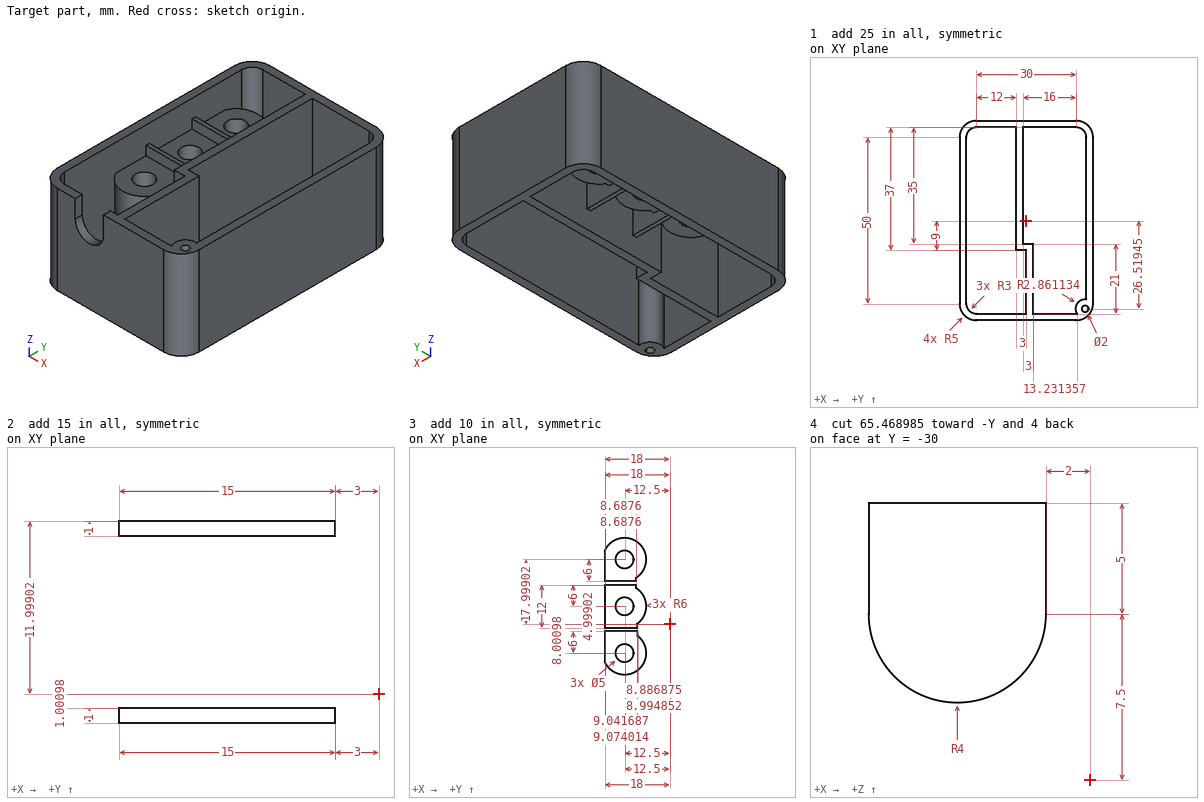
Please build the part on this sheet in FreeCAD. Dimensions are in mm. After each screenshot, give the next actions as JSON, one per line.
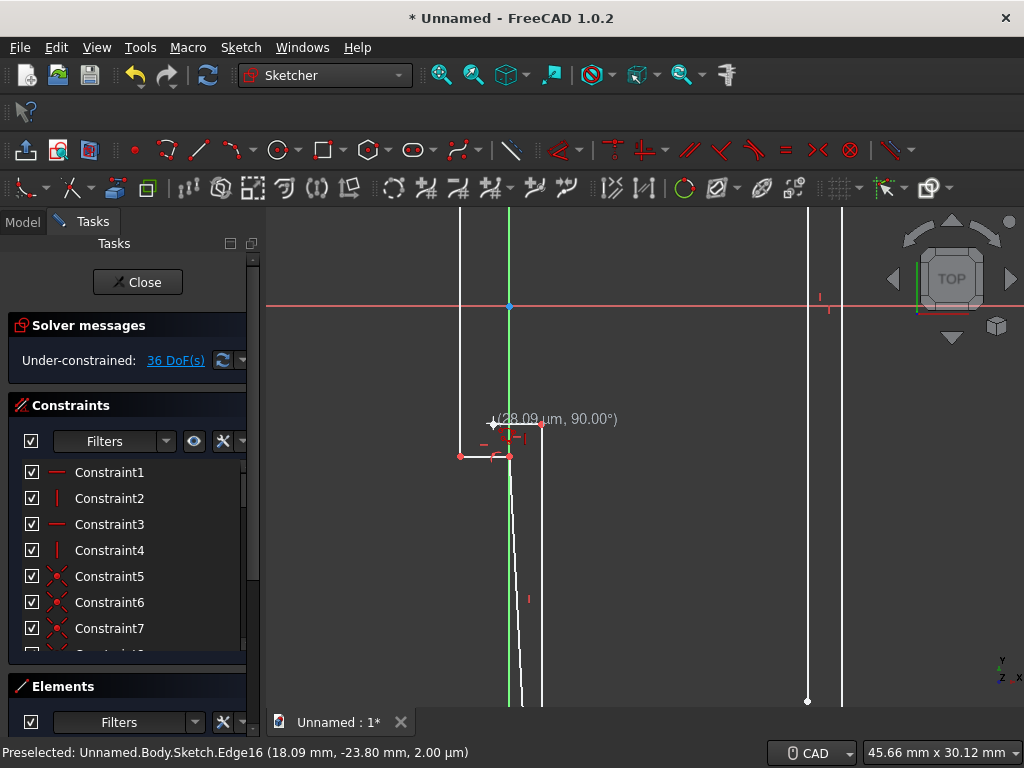
{"action": "scroll", "coordinate": [605, 522], "scroll_direction": "down", "scroll_amount": 6}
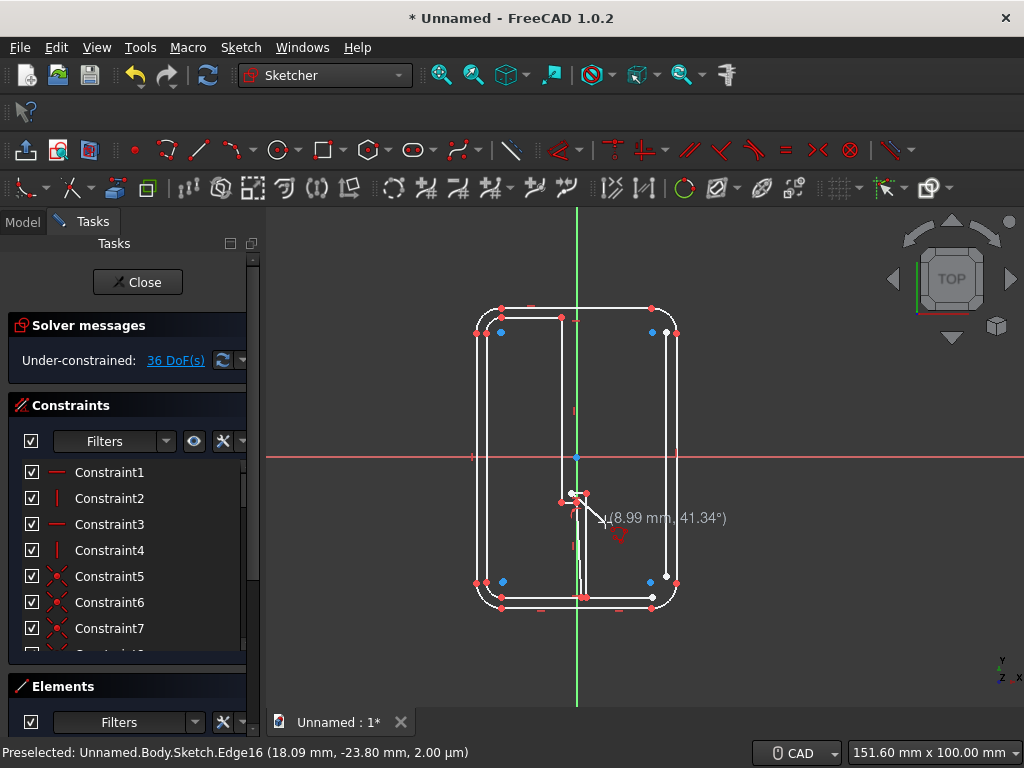
{"action": "scroll", "coordinate": [572, 317], "scroll_direction": "up", "scroll_amount": 6}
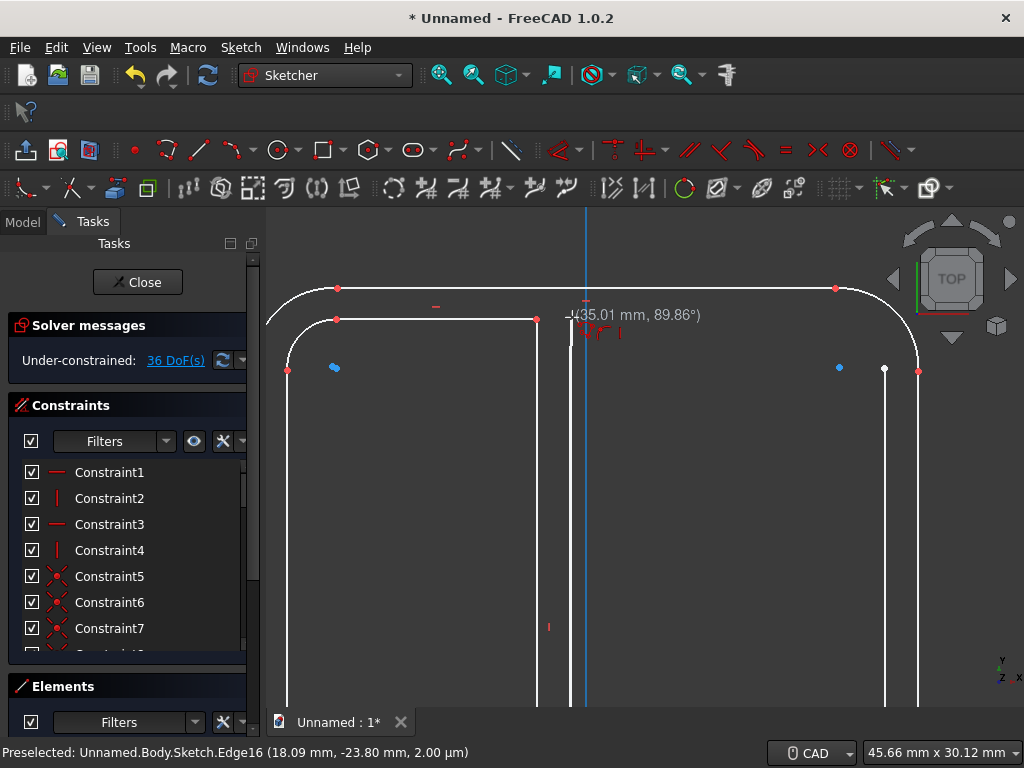
{"action": "left_click", "coordinate": [570, 318]}
{"action": "left_click", "coordinate": [835, 318]}
{"action": "right_click", "coordinate": [835, 318]}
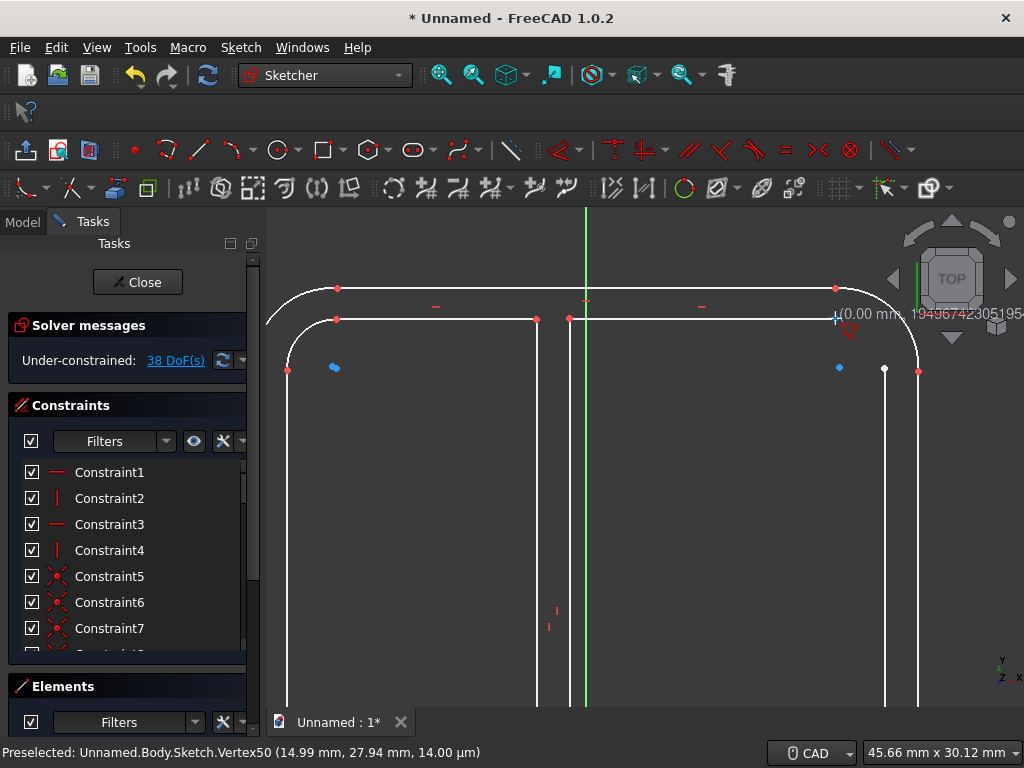
{"action": "left_click", "coordinate": [232, 150]}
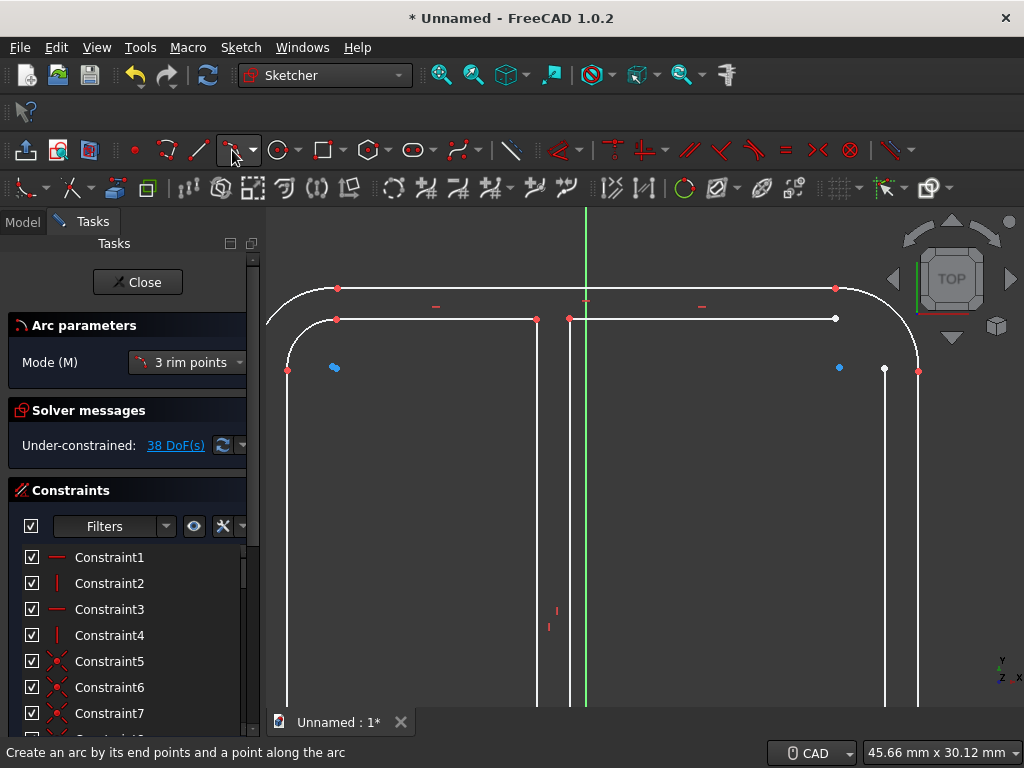
{"action": "scroll", "coordinate": [572, 317], "scroll_direction": "down", "scroll_amount": 6}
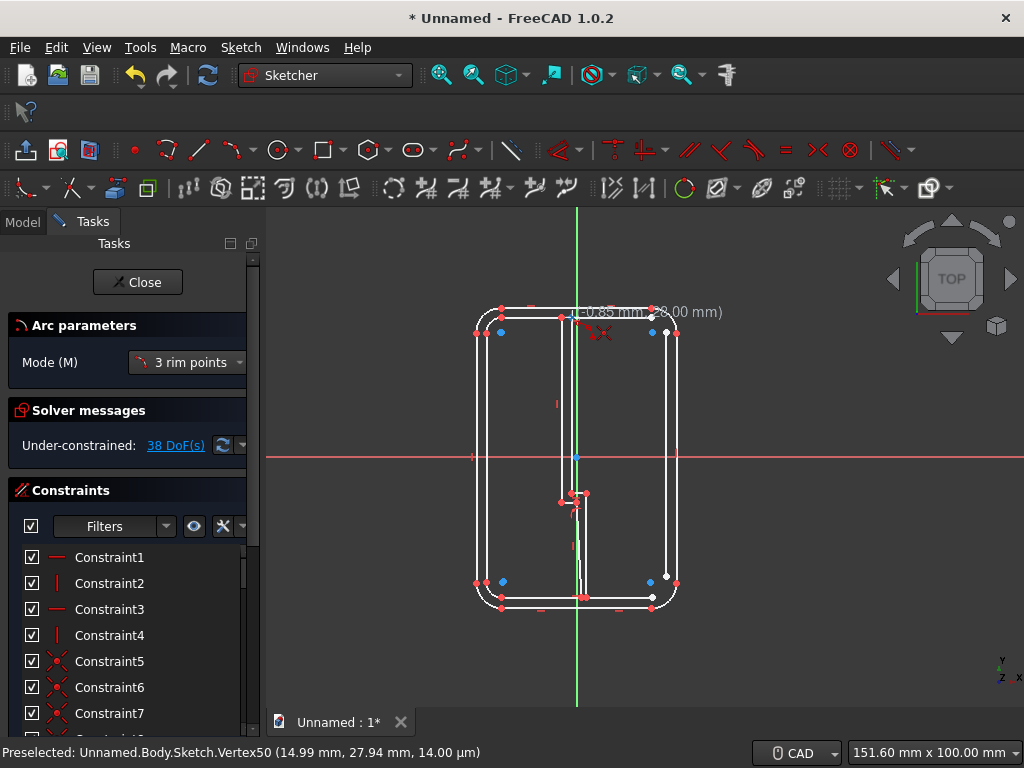
{"action": "scroll", "coordinate": [667, 576], "scroll_direction": "up", "scroll_amount": 3}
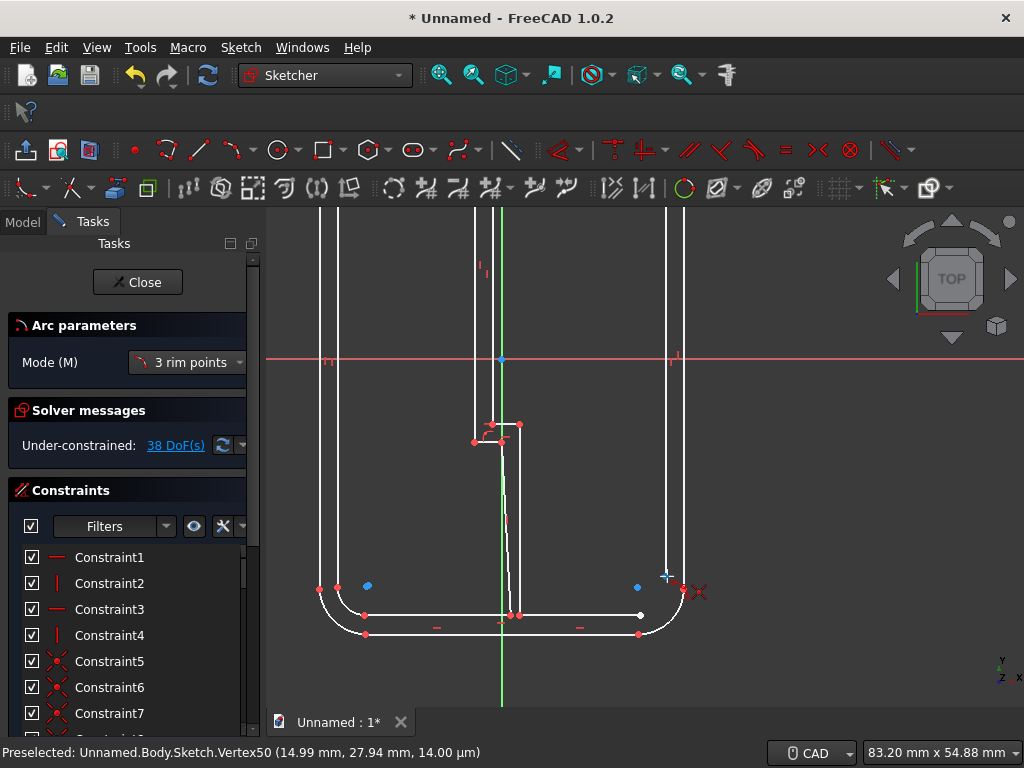
{"action": "left_click", "coordinate": [666, 576]}
{"action": "left_click", "coordinate": [641, 615]}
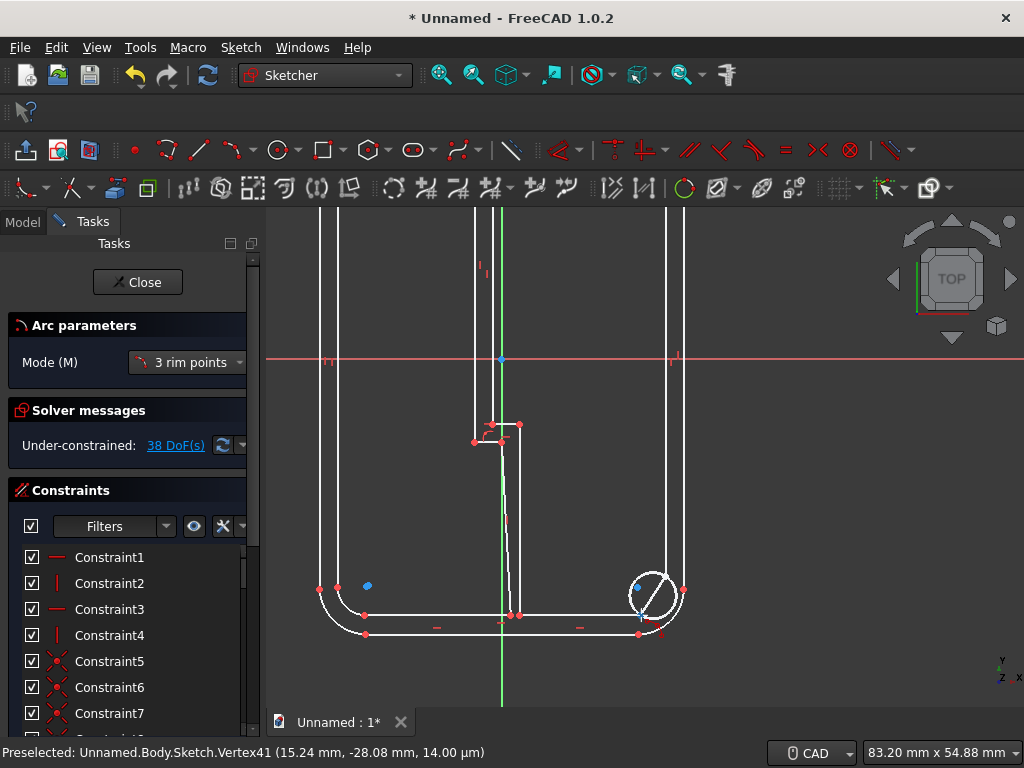
{"action": "scroll", "coordinate": [649, 579], "scroll_direction": "up", "scroll_amount": 2}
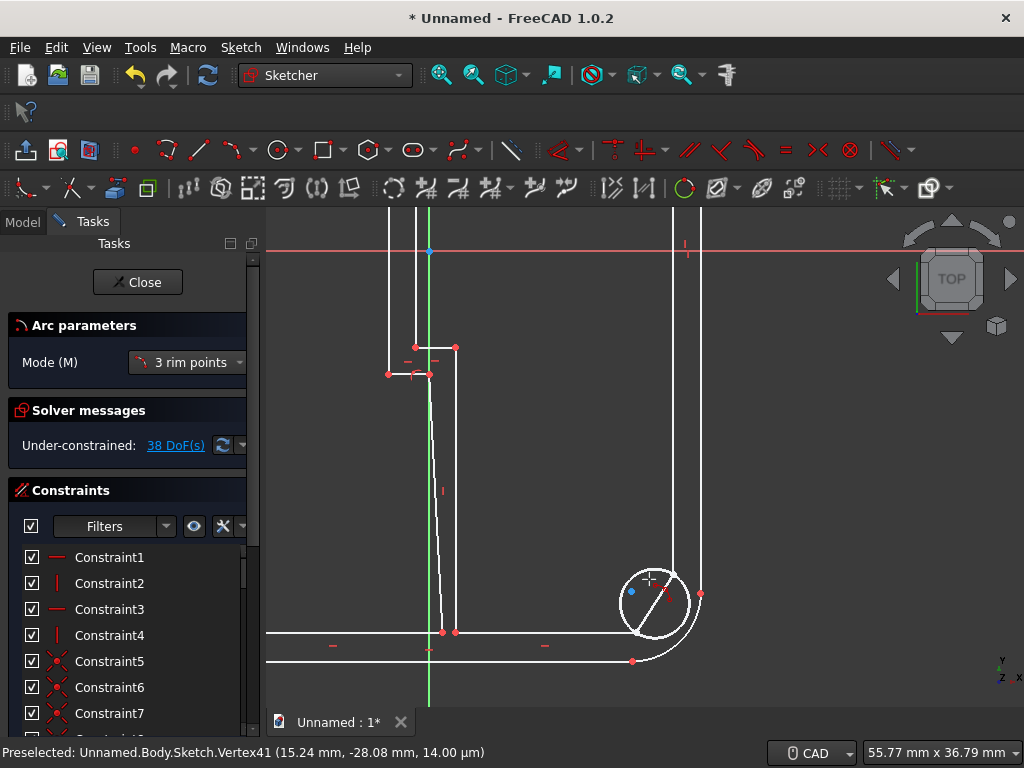
{"action": "left_click", "coordinate": [649, 578]}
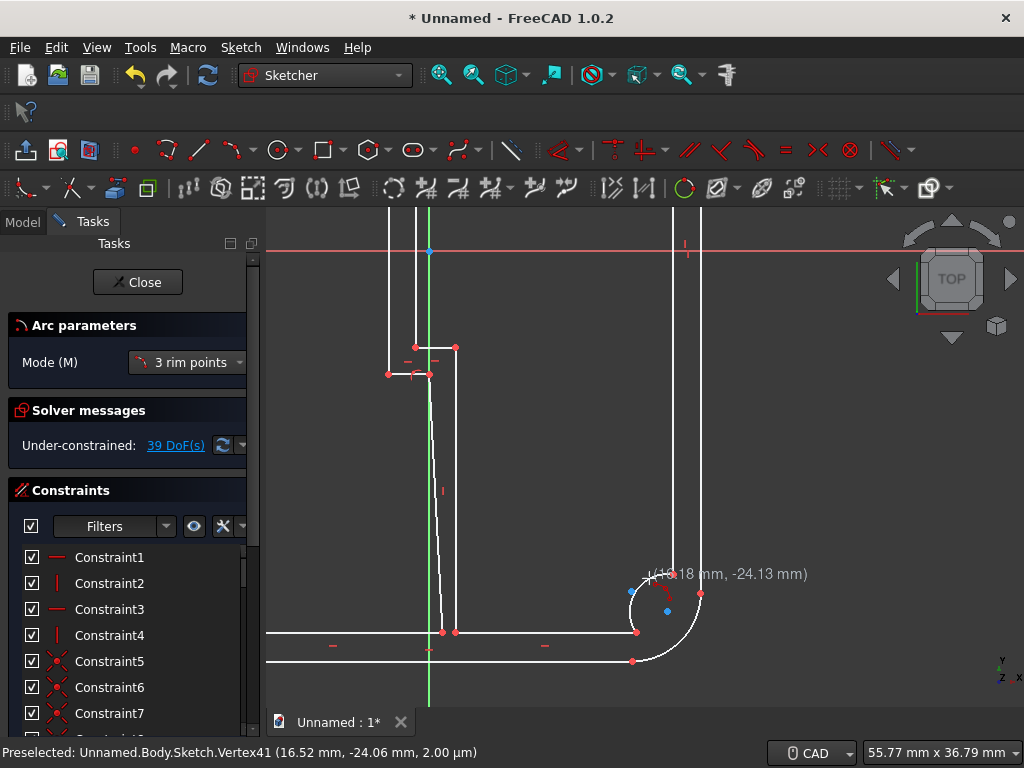
{"action": "scroll", "coordinate": [662, 577], "scroll_direction": "down", "scroll_amount": 5}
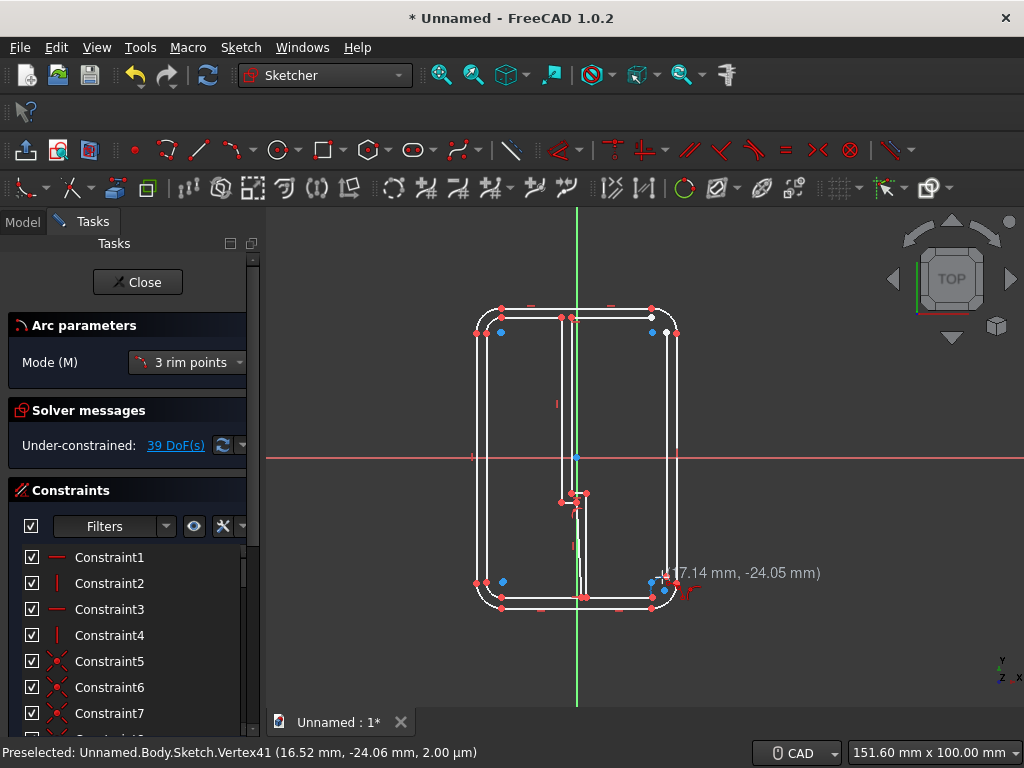
{"action": "scroll", "coordinate": [652, 318], "scroll_direction": "up", "scroll_amount": 3}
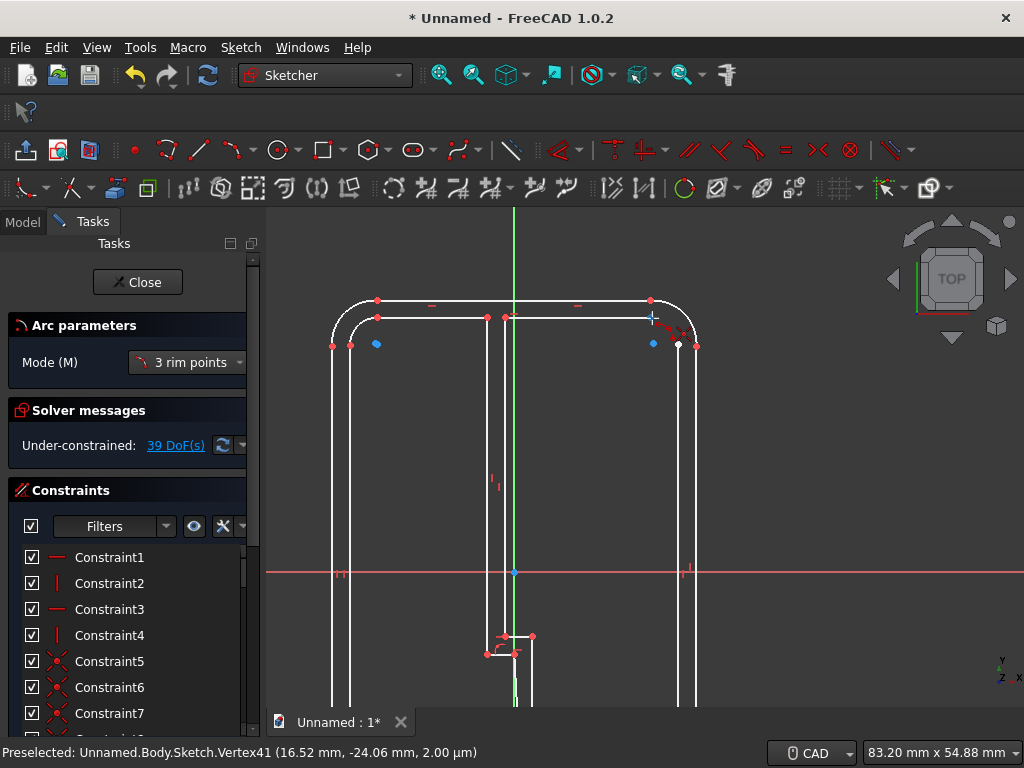
{"action": "left_click", "coordinate": [651, 318]}
{"action": "left_click", "coordinate": [678, 345]}